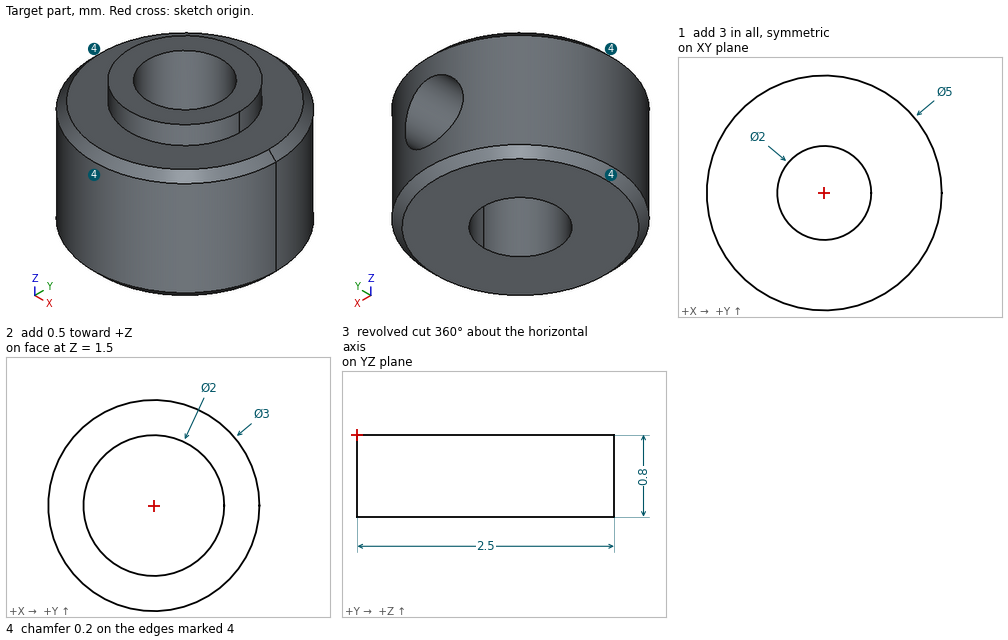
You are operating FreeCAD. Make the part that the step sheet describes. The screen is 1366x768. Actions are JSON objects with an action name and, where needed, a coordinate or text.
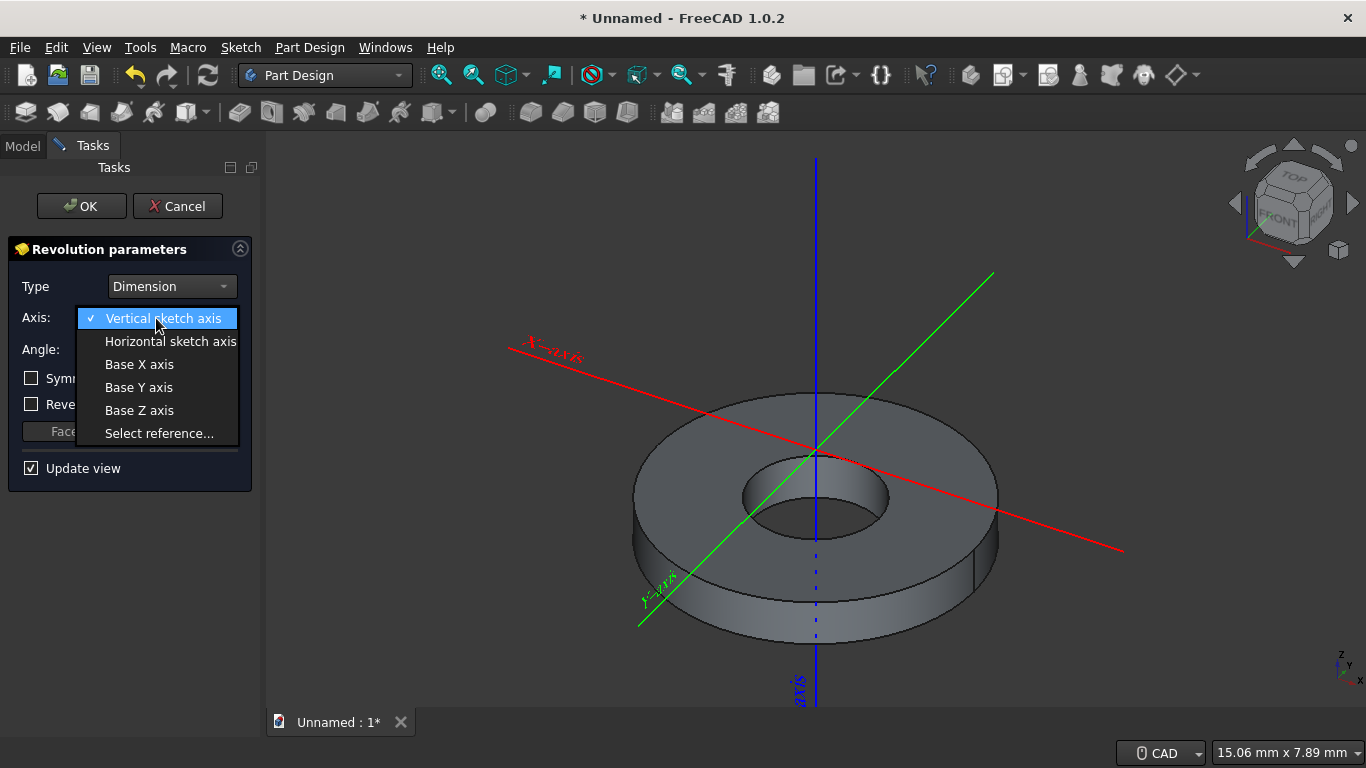
{"action": "left_click", "coordinate": [156, 342]}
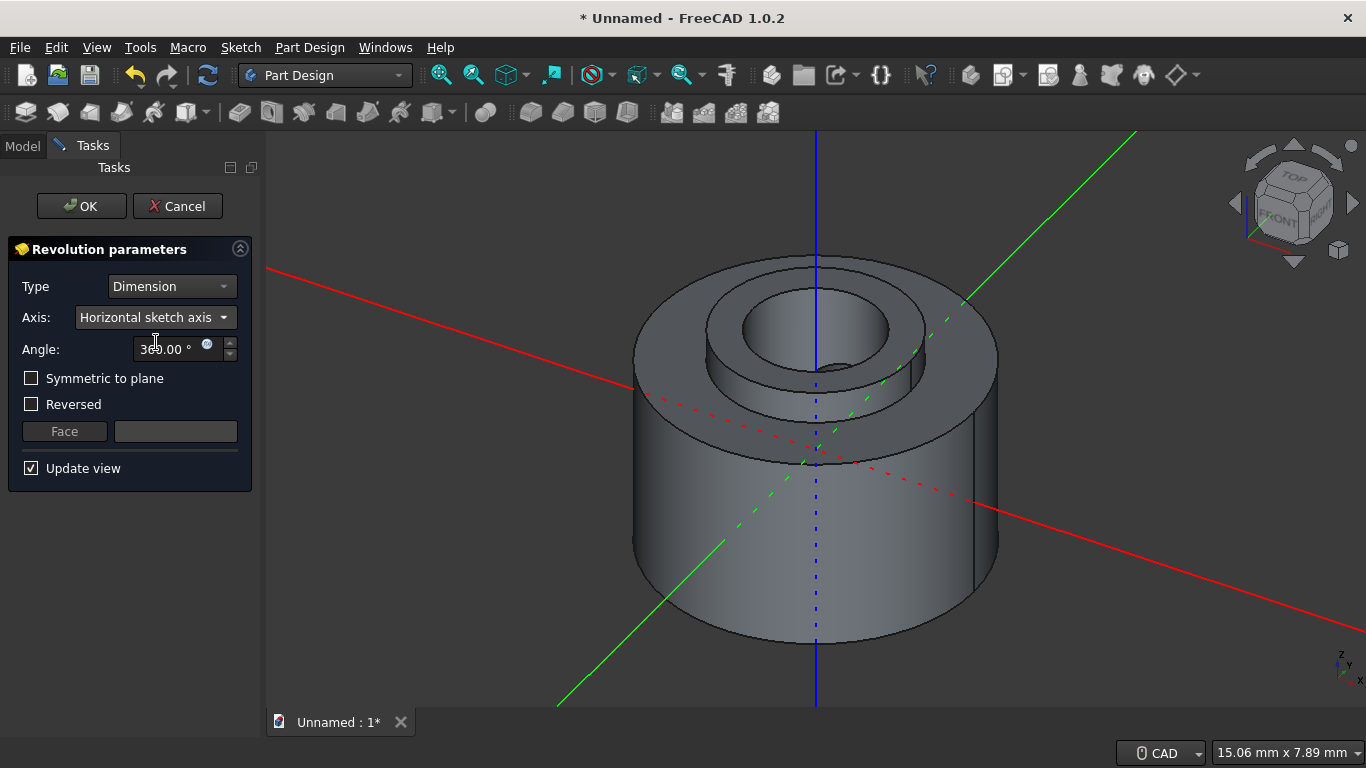
{"action": "left_click", "coordinate": [82, 206]}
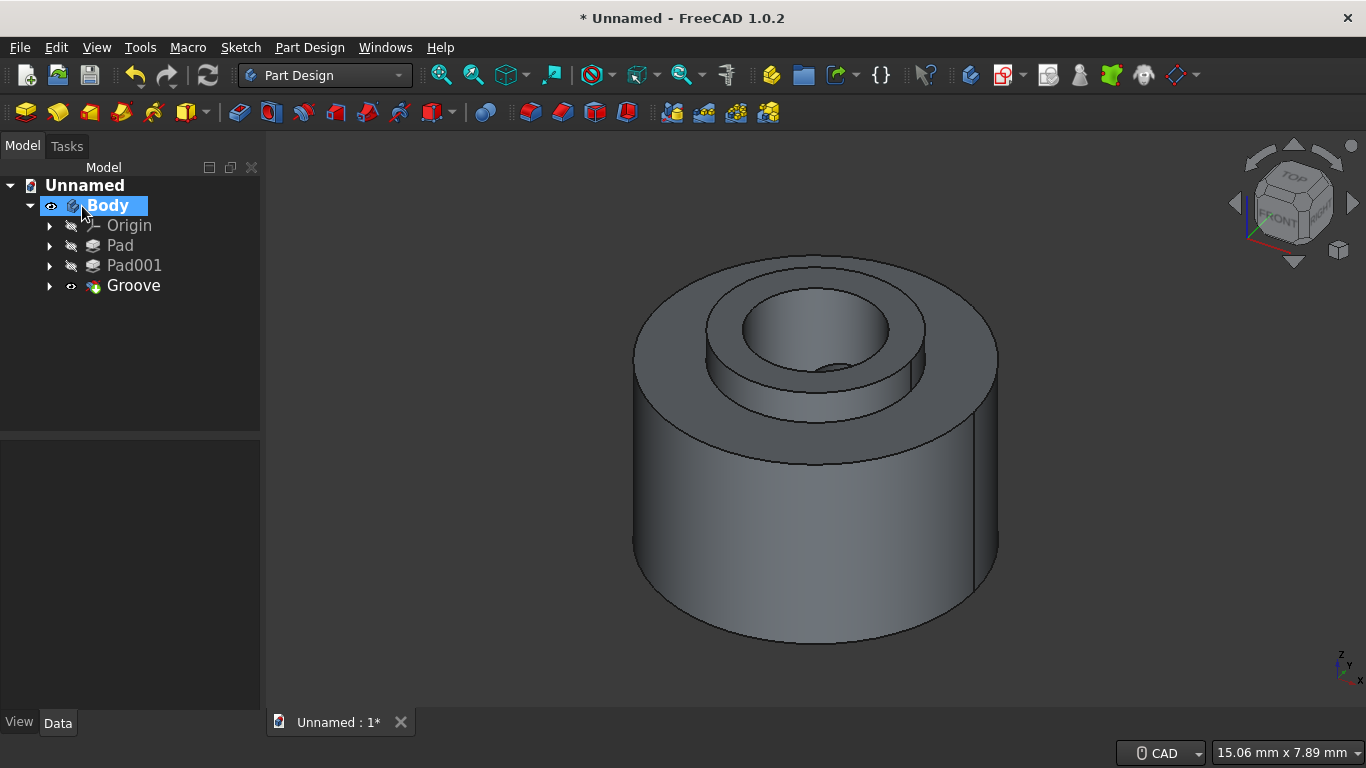
{"action": "left_click", "coordinate": [634, 370]}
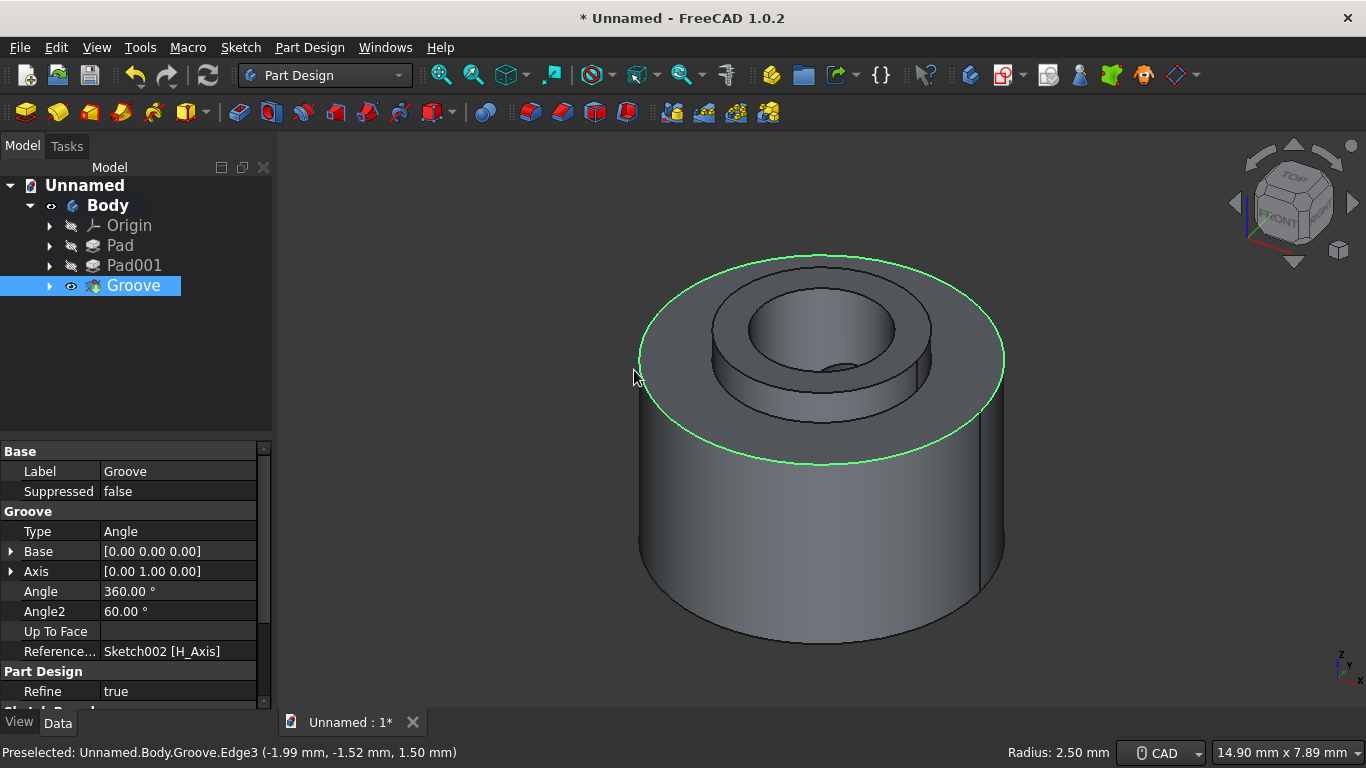
{"action": "key", "text": "0"}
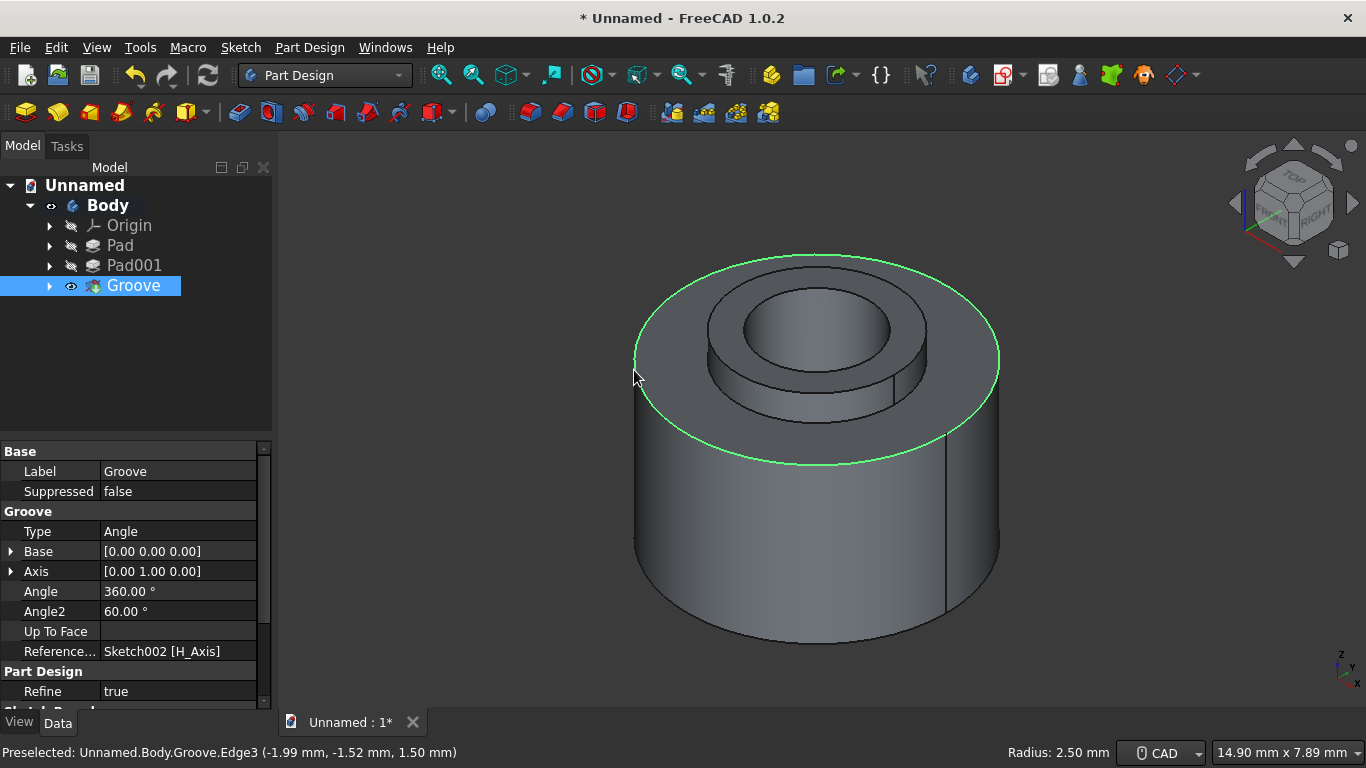
{"action": "key", "text": "2"}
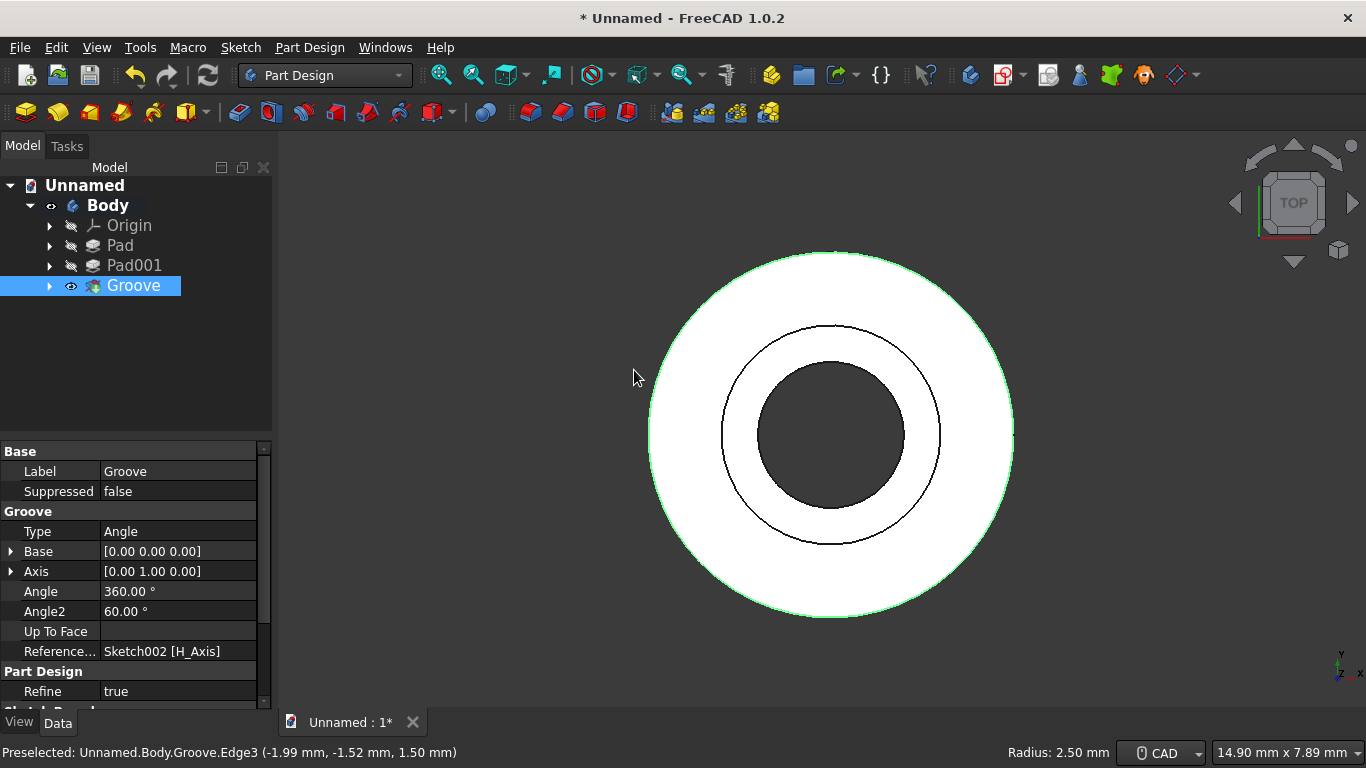
{"action": "key", "text": "1"}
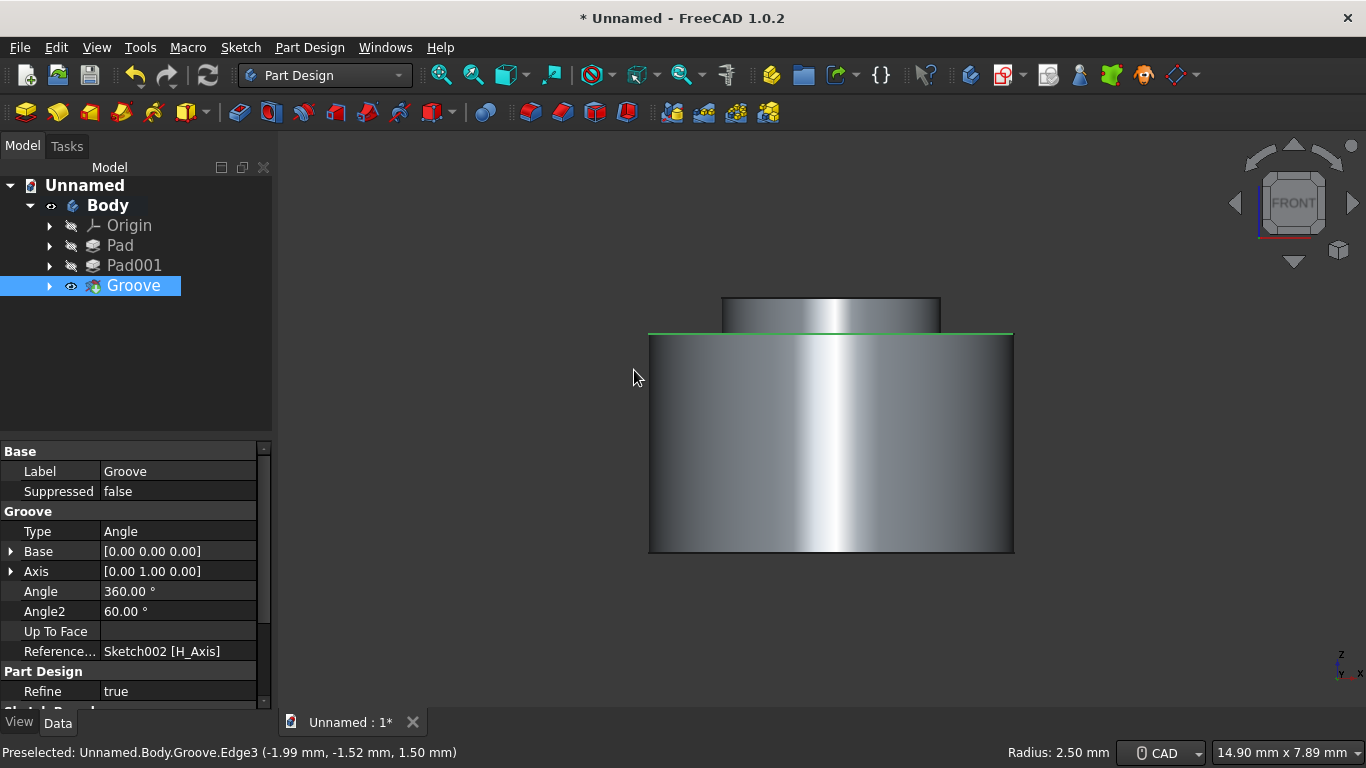
{"action": "left_click", "coordinate": [442, 76]}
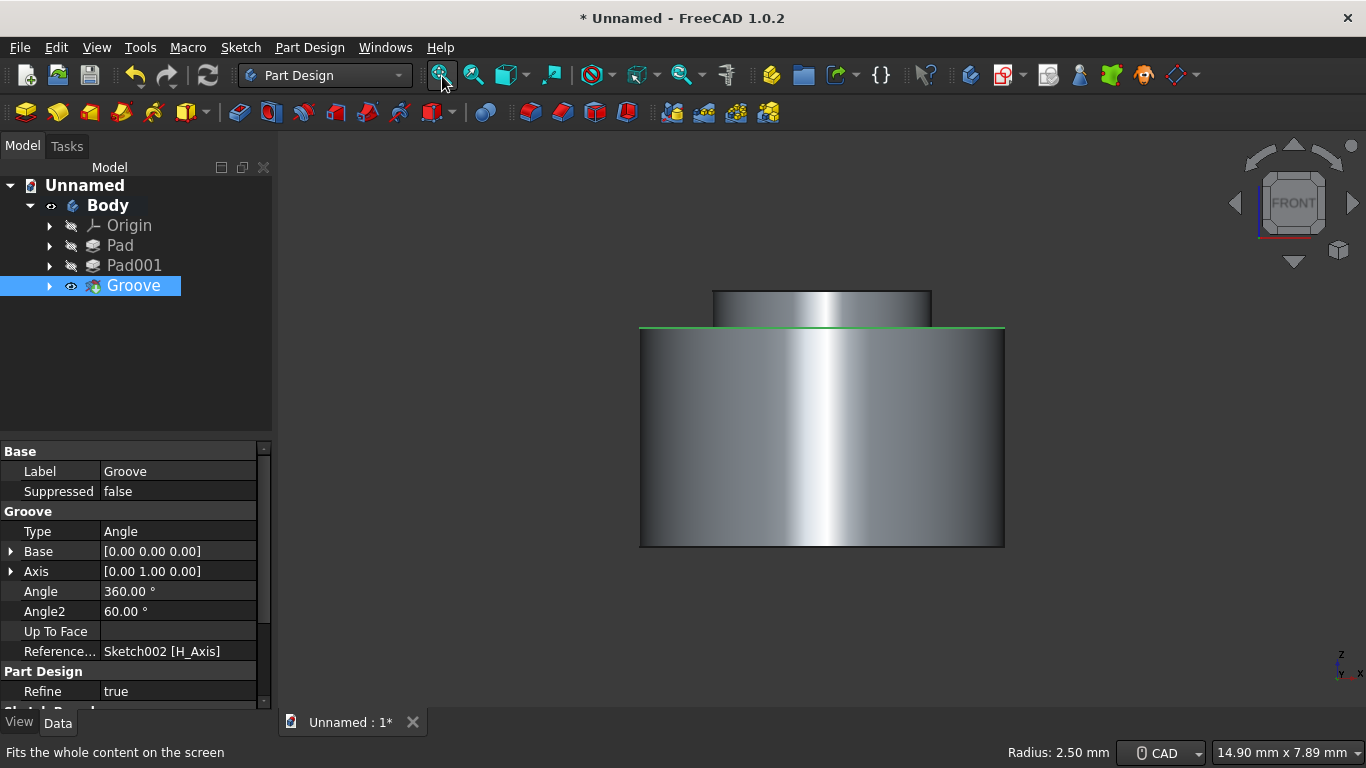
{"action": "left_click", "coordinate": [674, 546], "text": "ctrl"}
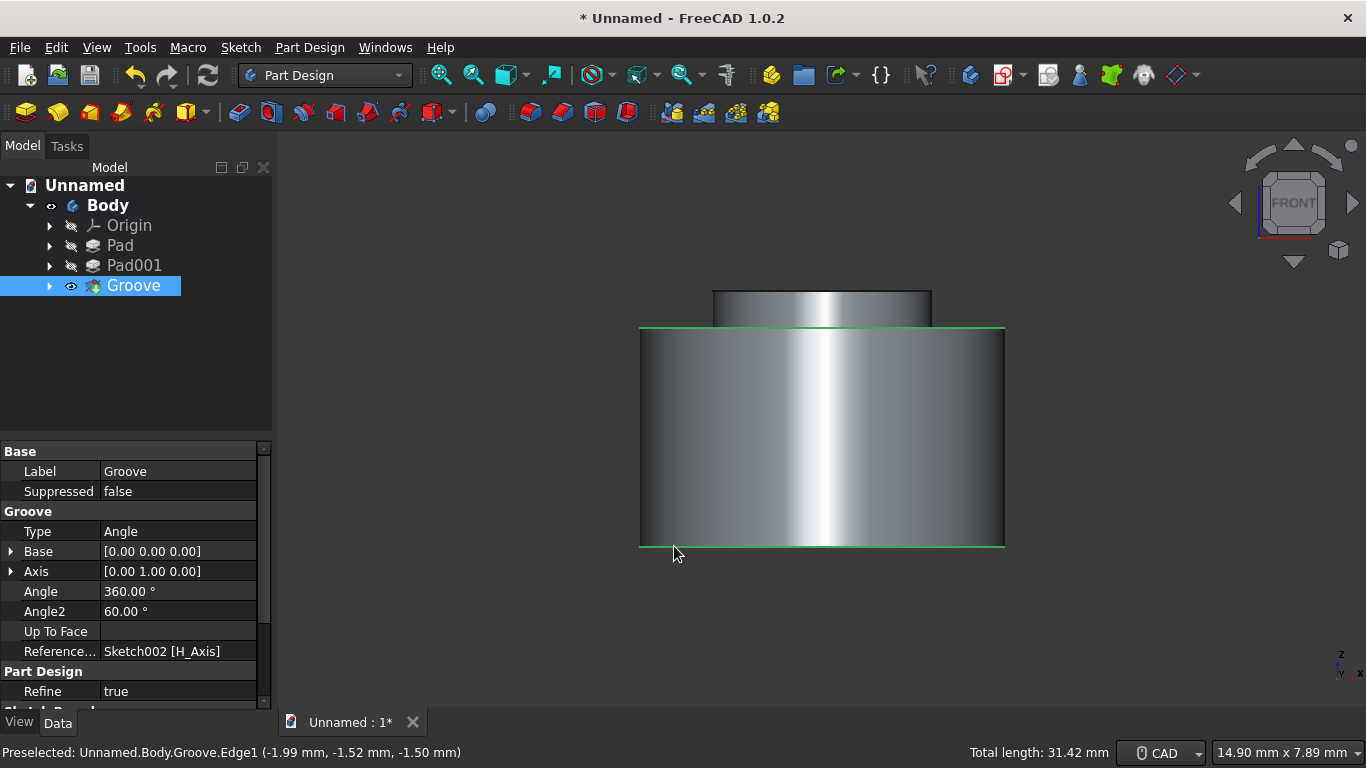
{"action": "left_click", "coordinate": [564, 112]}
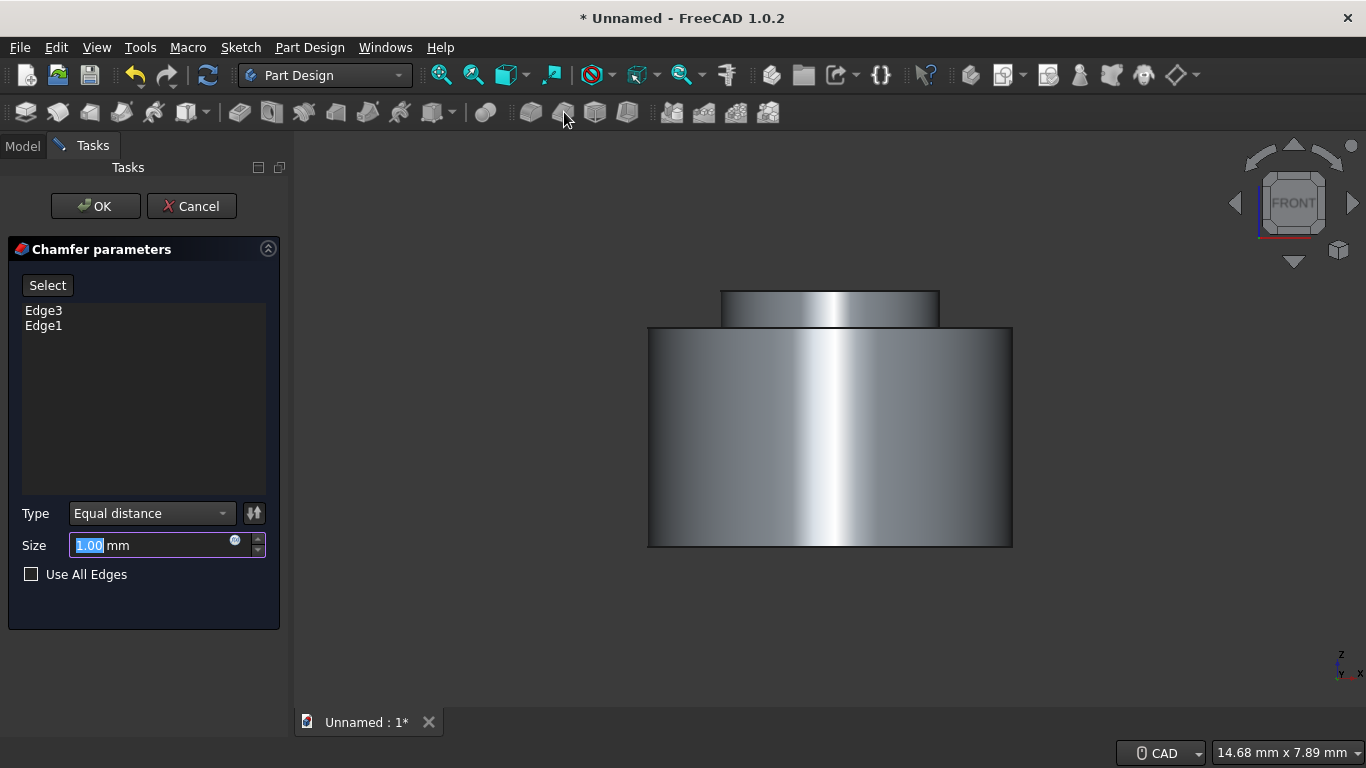
{"action": "type", "text": "0.2"}
{"action": "key", "text": "Tab"}